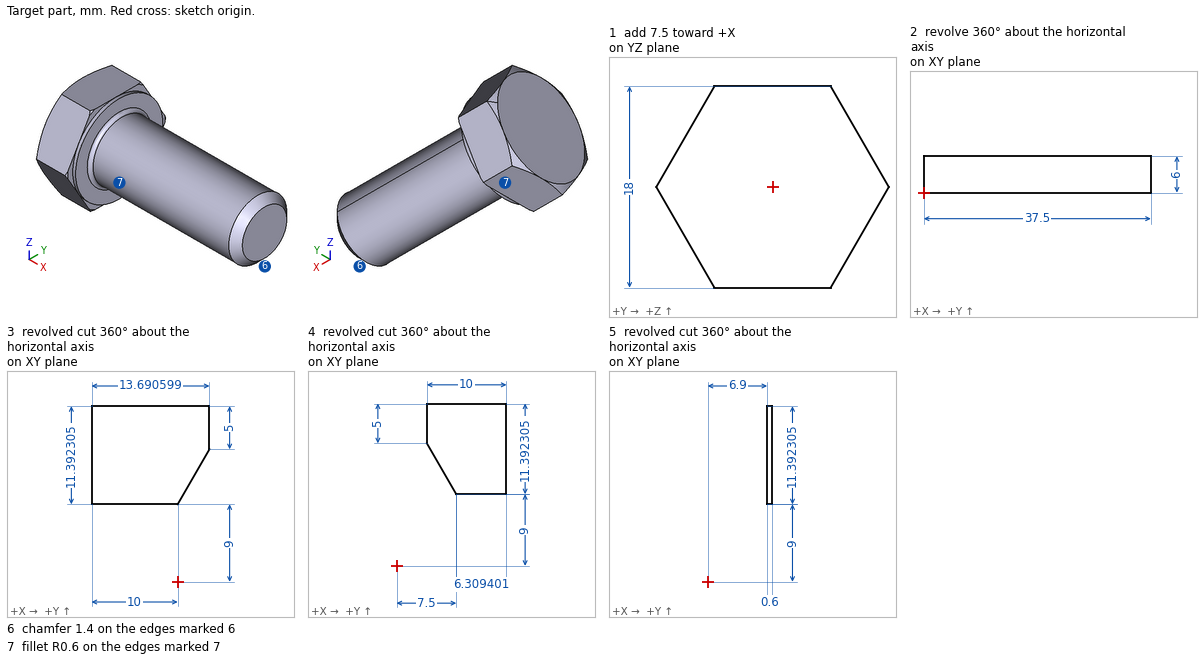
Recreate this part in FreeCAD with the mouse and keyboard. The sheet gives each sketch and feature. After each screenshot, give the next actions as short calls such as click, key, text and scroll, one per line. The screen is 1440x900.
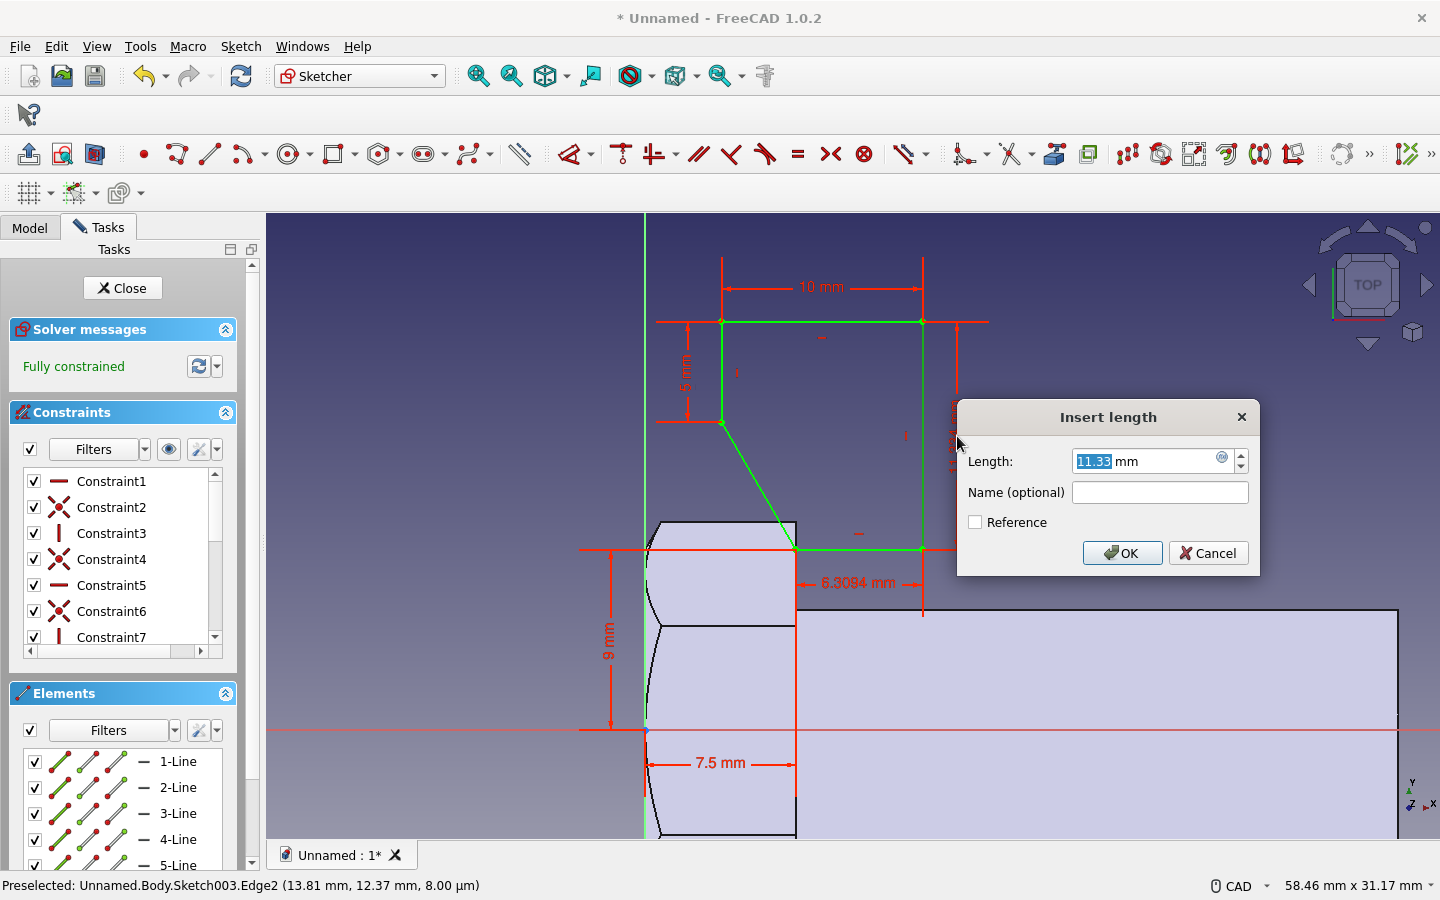
text(11.392305)
key(Return)
key(Escape)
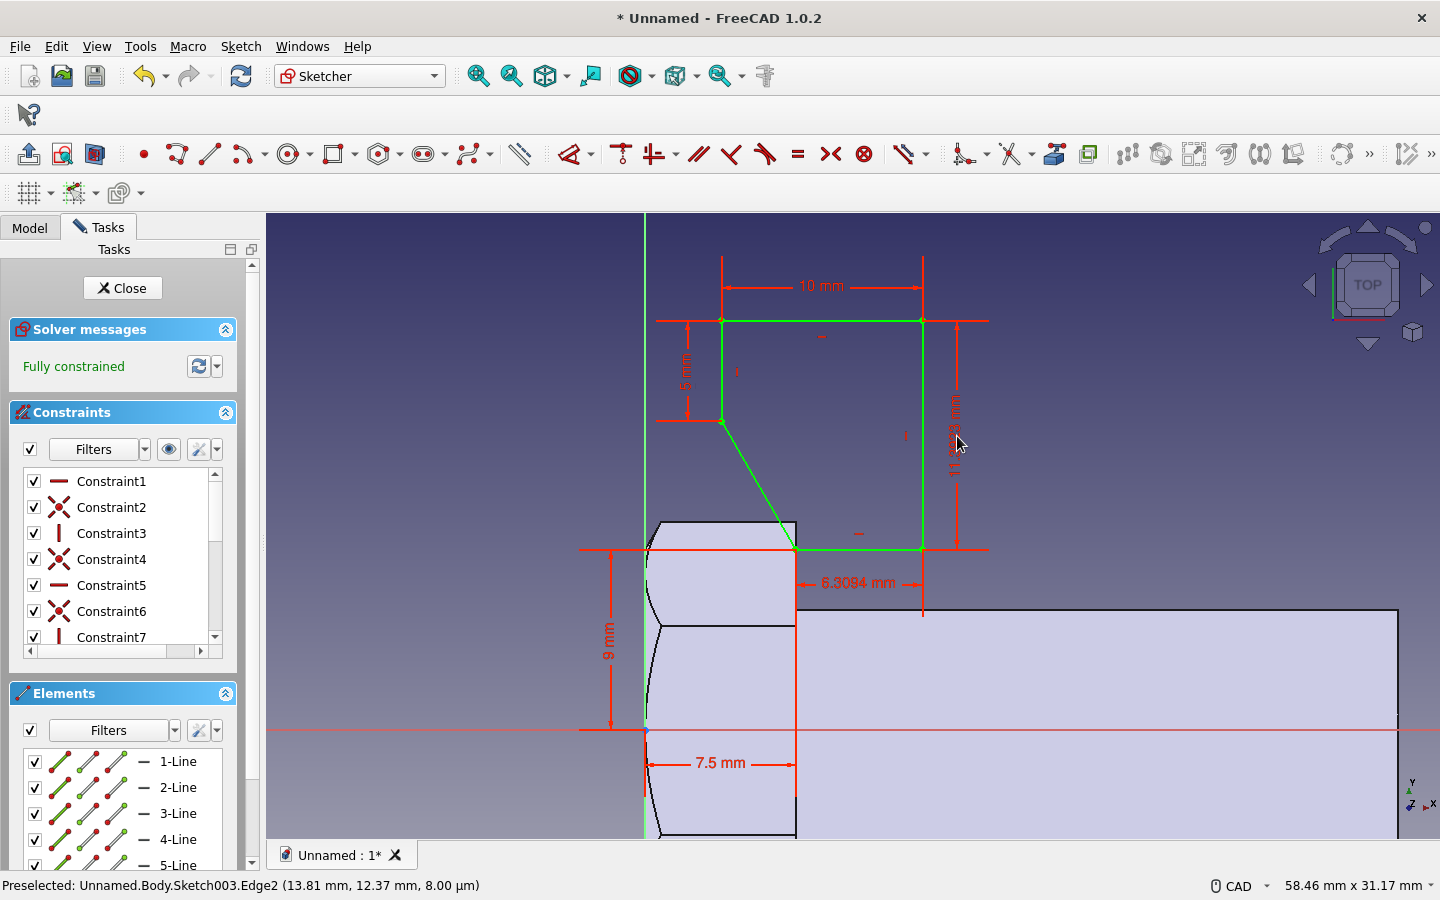
click(123, 288)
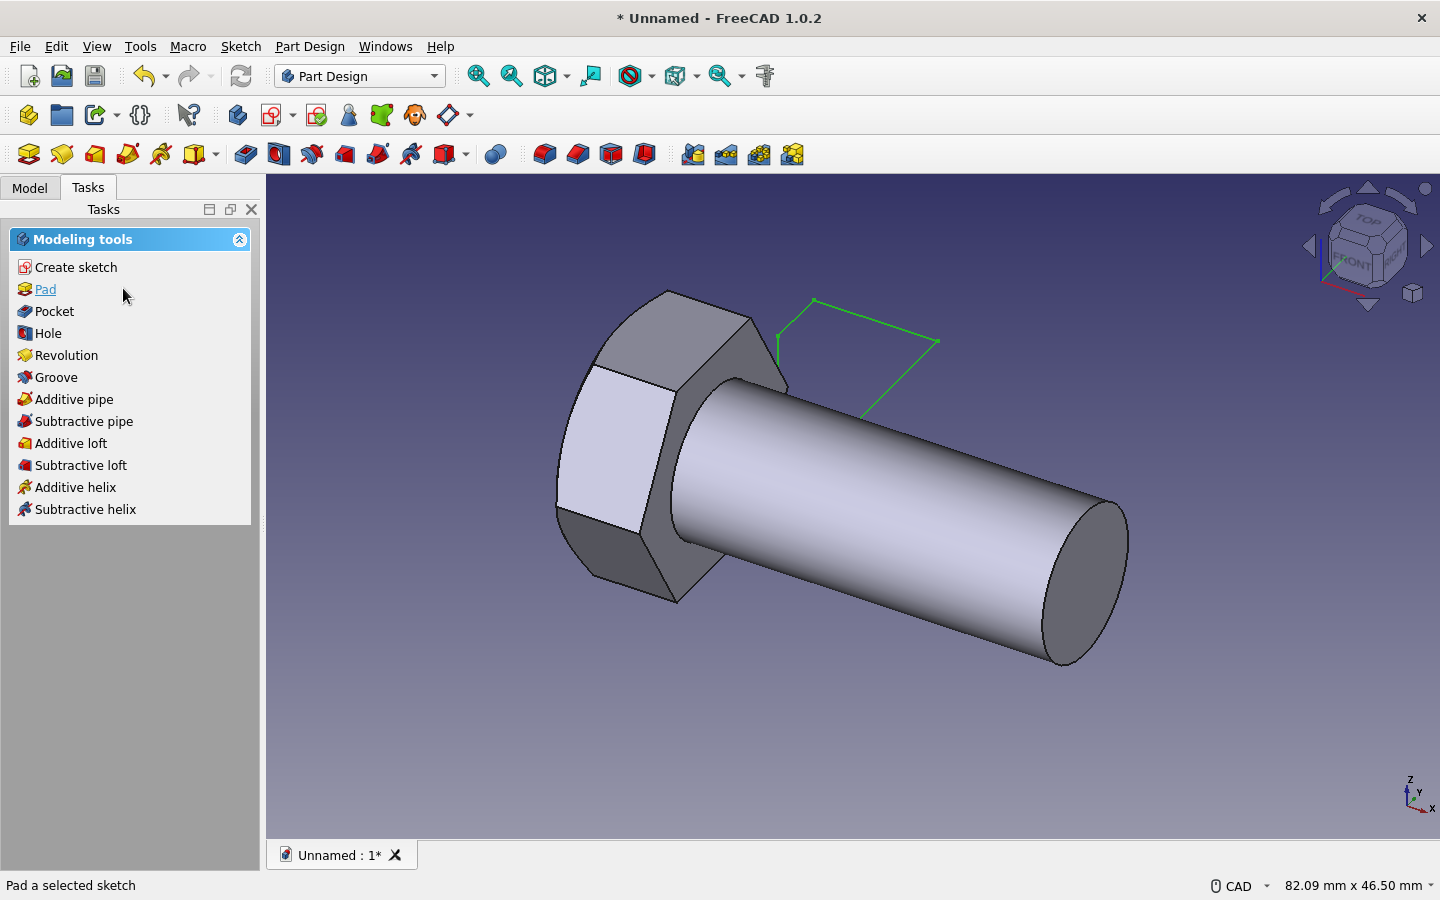
click(312, 154)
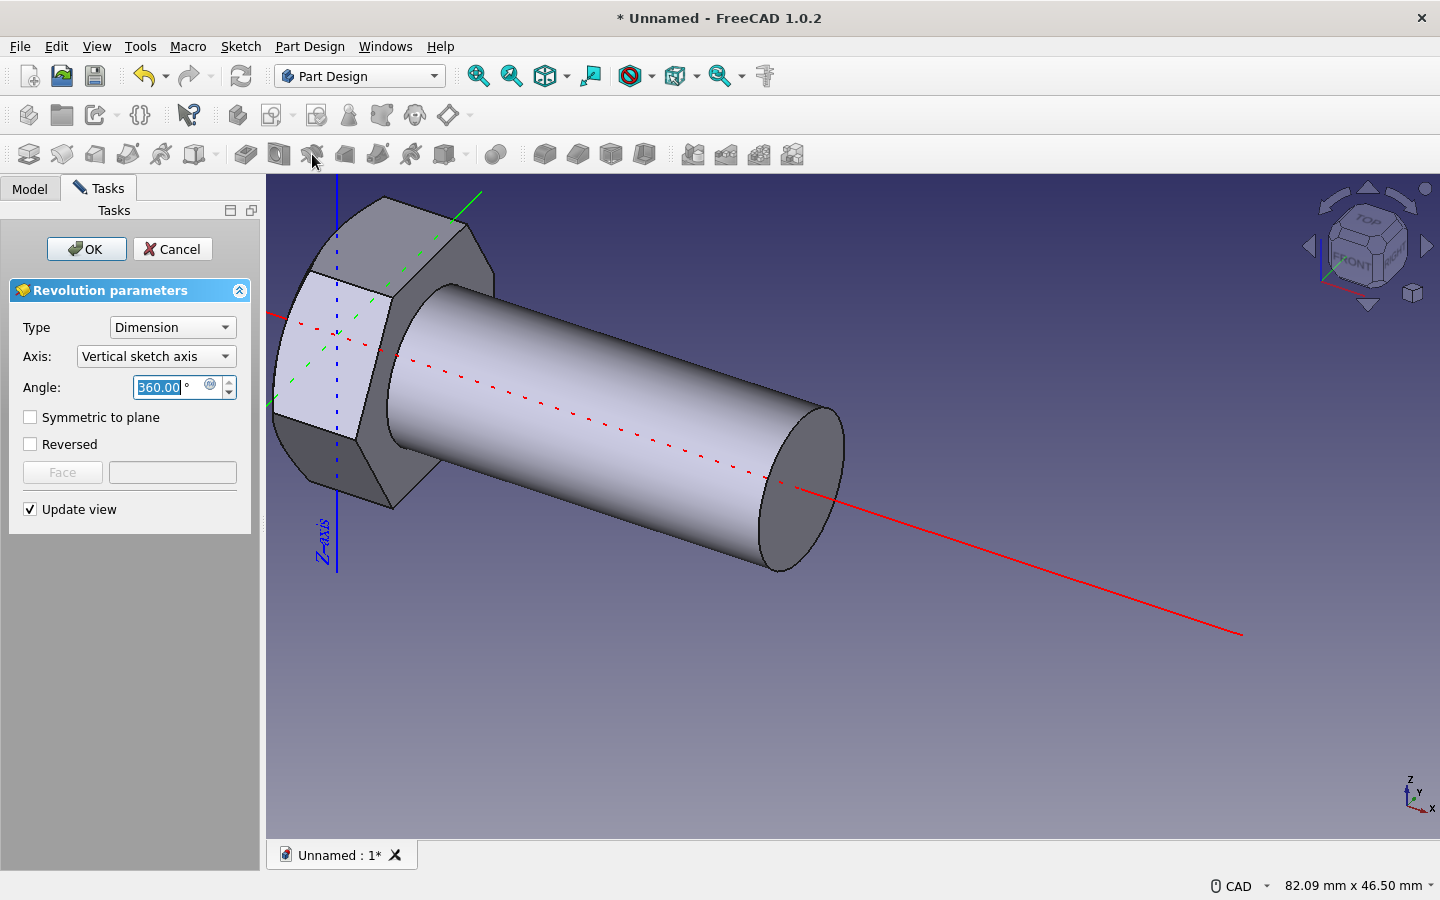
click(157, 356)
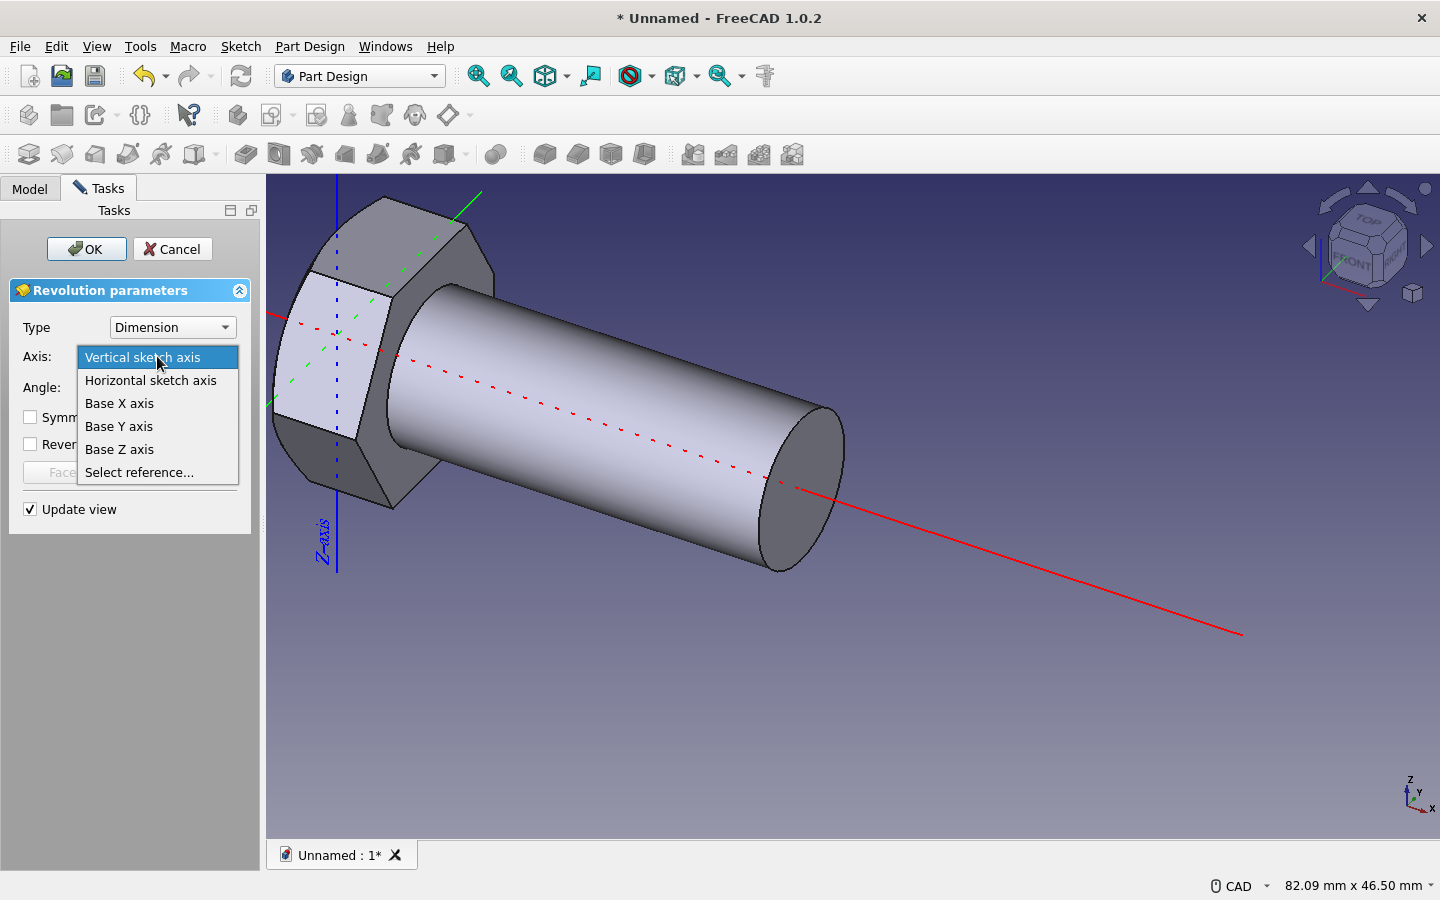
click(156, 380)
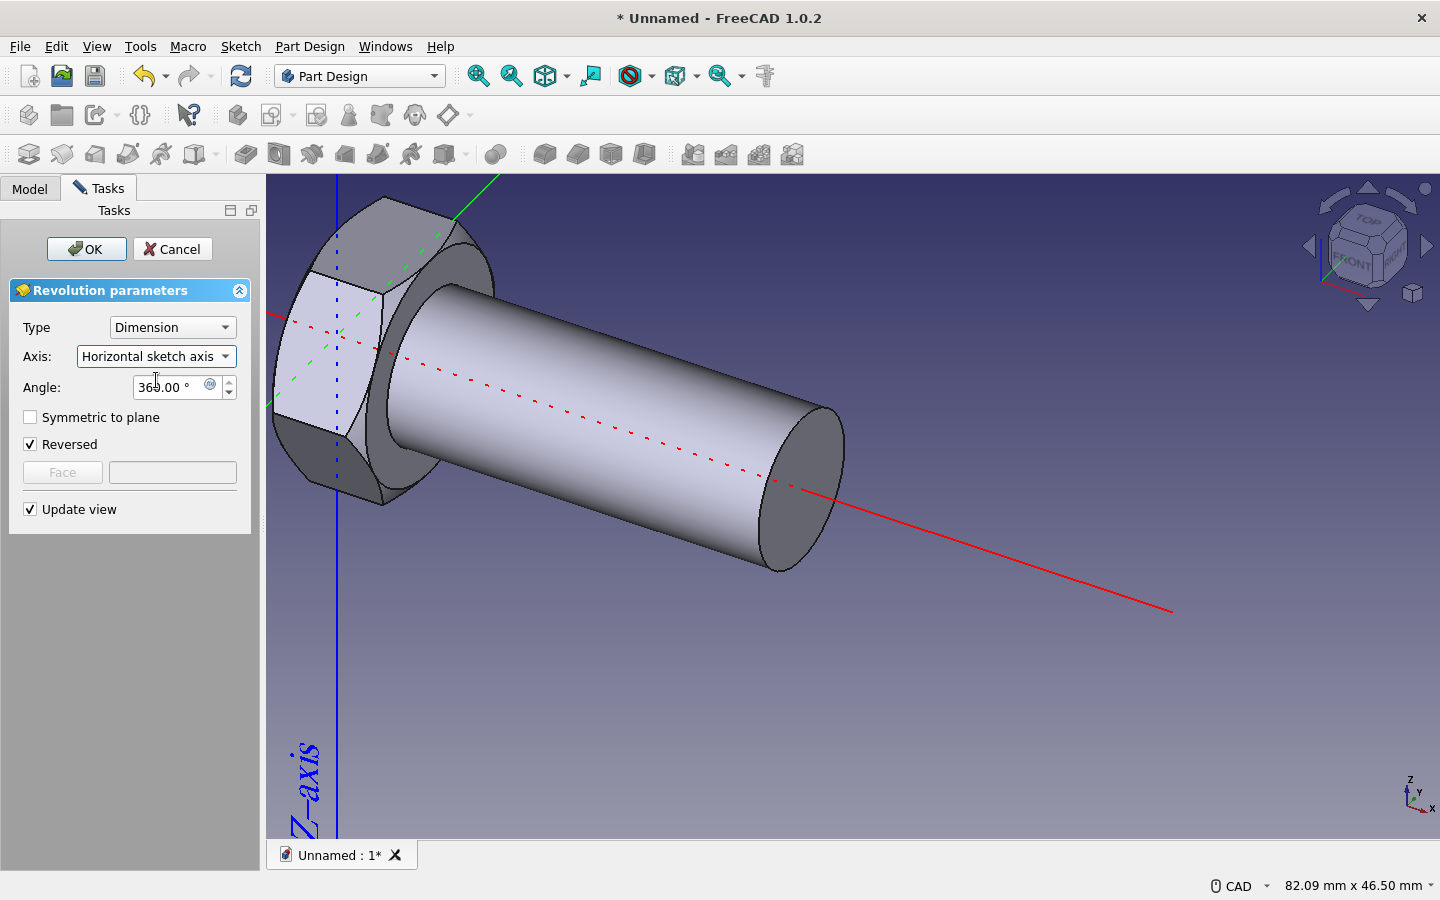
click(87, 249)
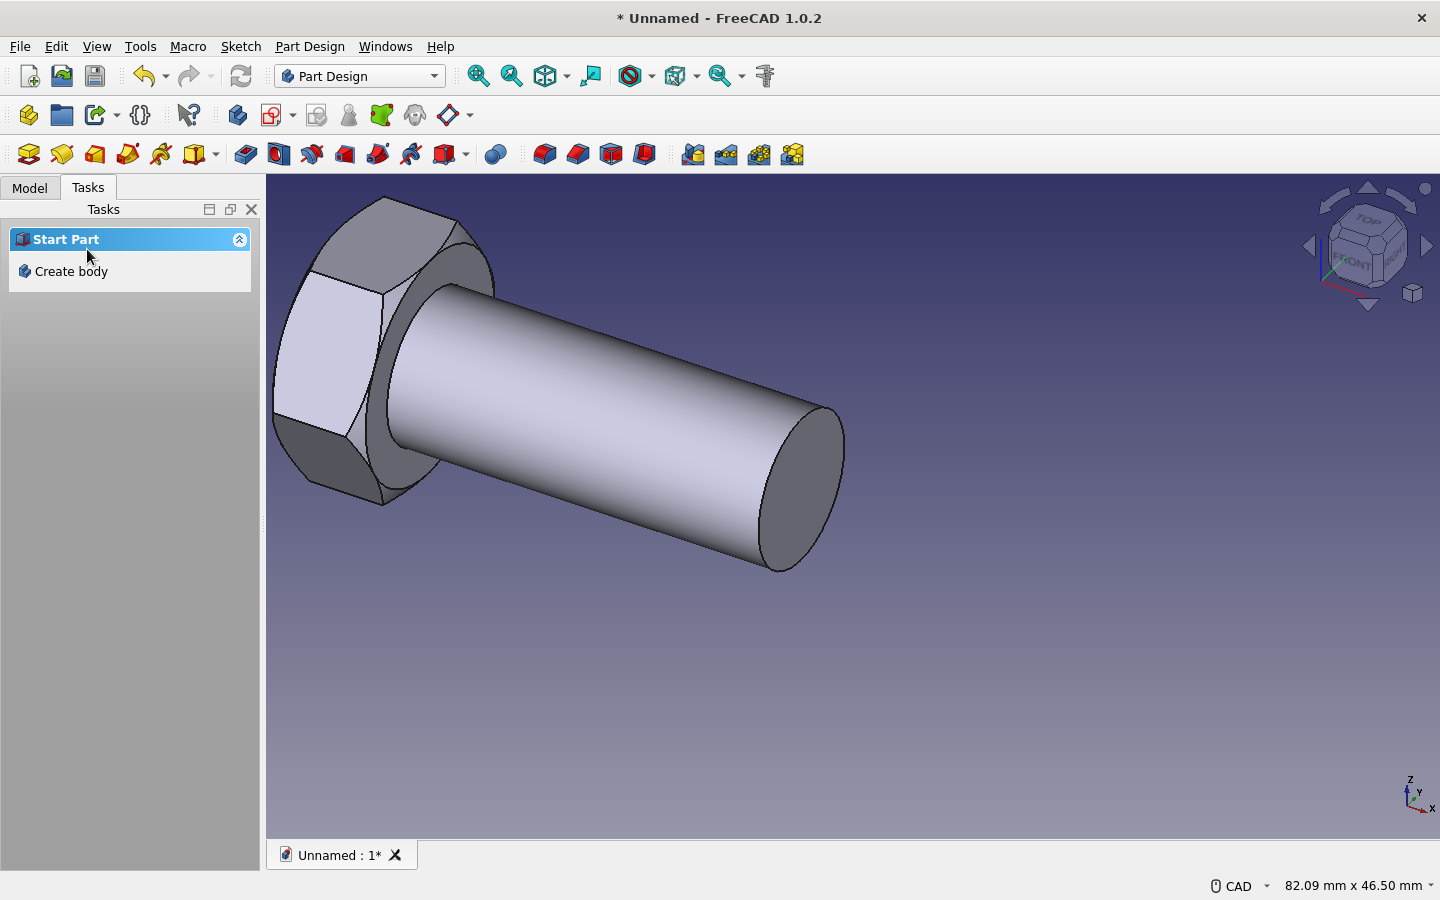
click(479, 76)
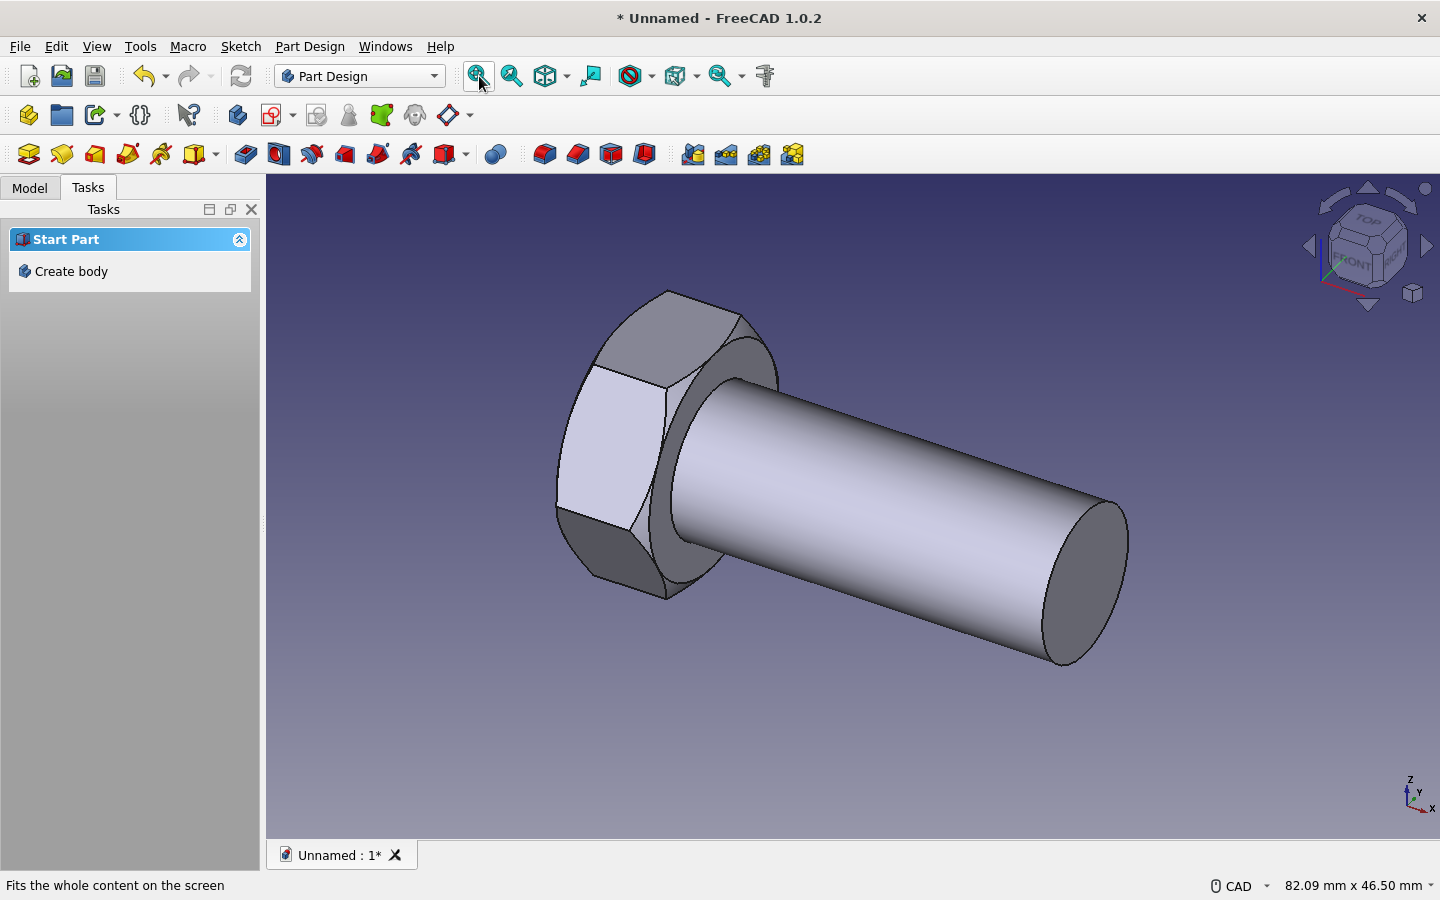
click(270, 116)